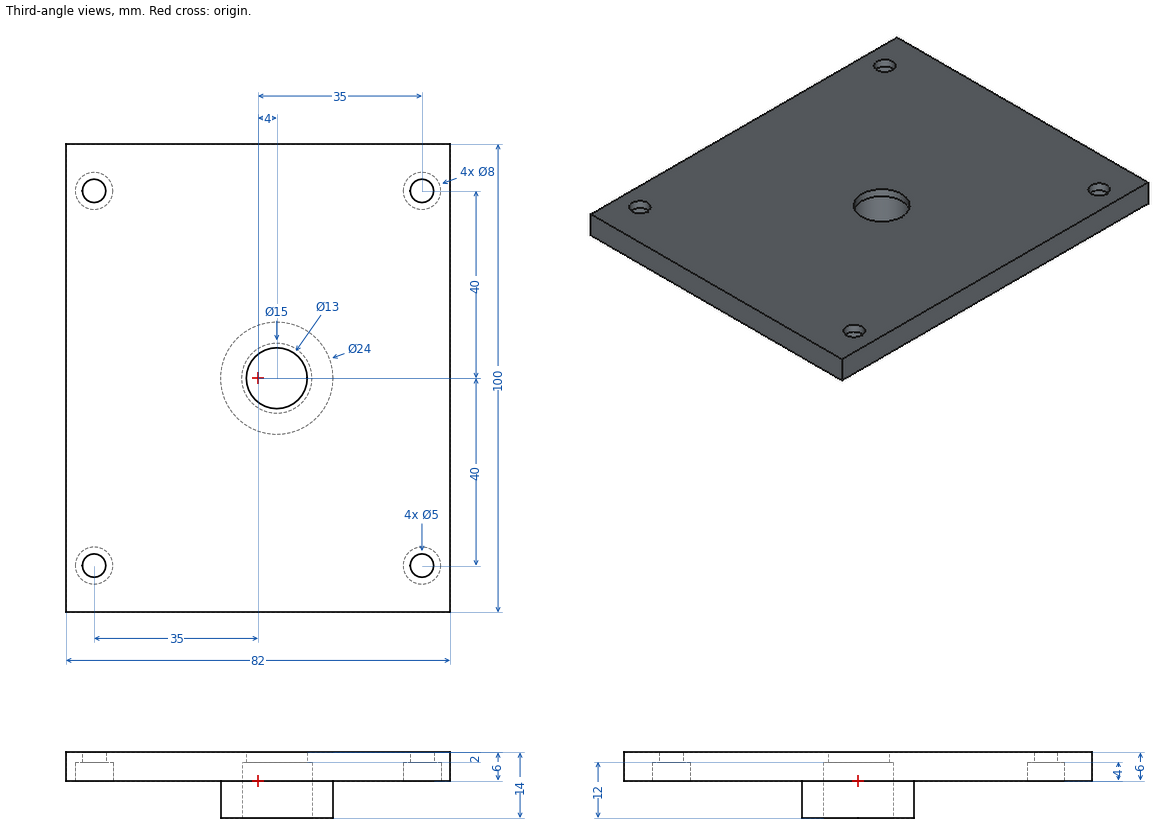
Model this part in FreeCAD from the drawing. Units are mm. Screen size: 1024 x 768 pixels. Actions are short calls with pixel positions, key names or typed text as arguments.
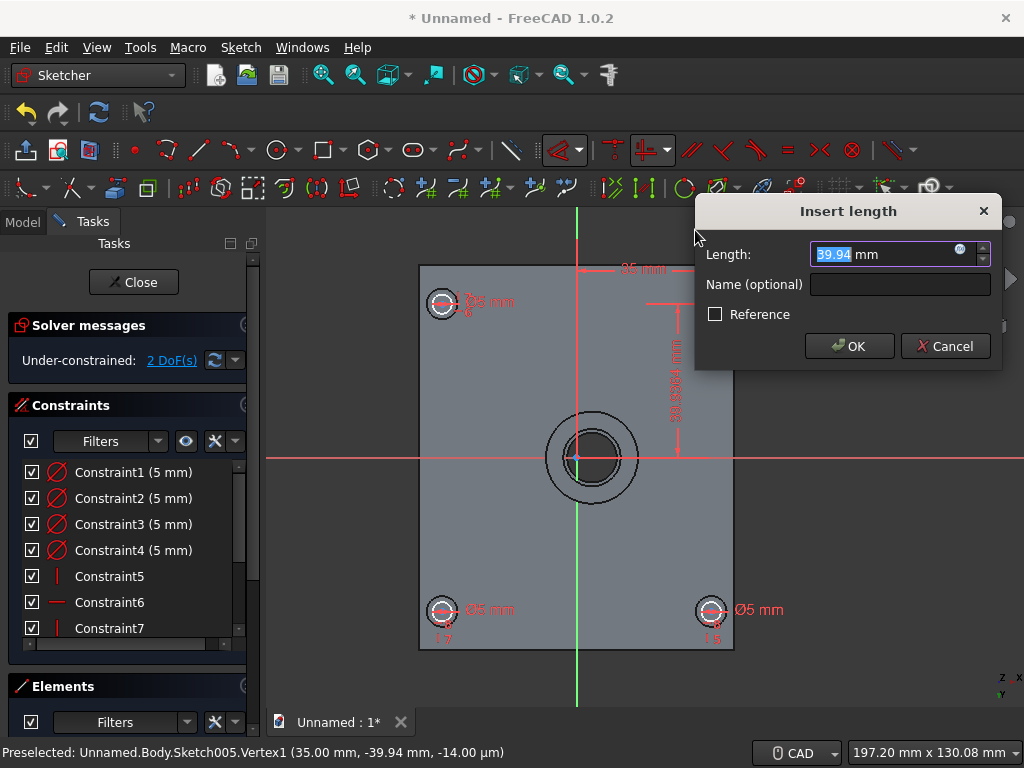
text(40)
key(Return)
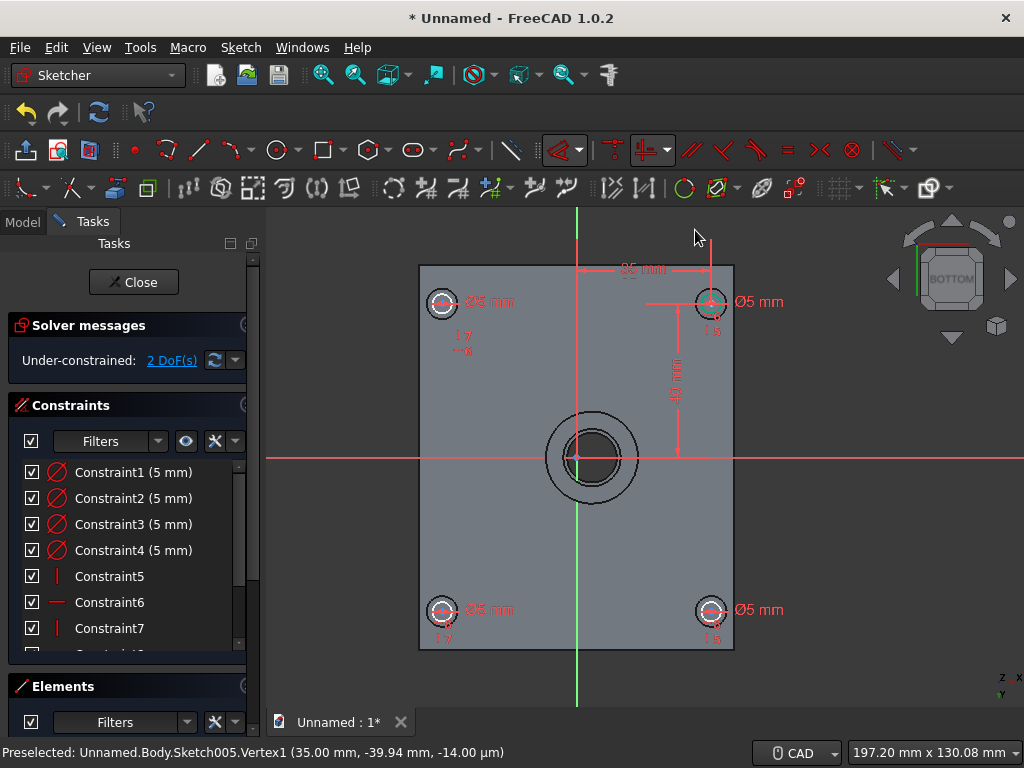
click(711, 612)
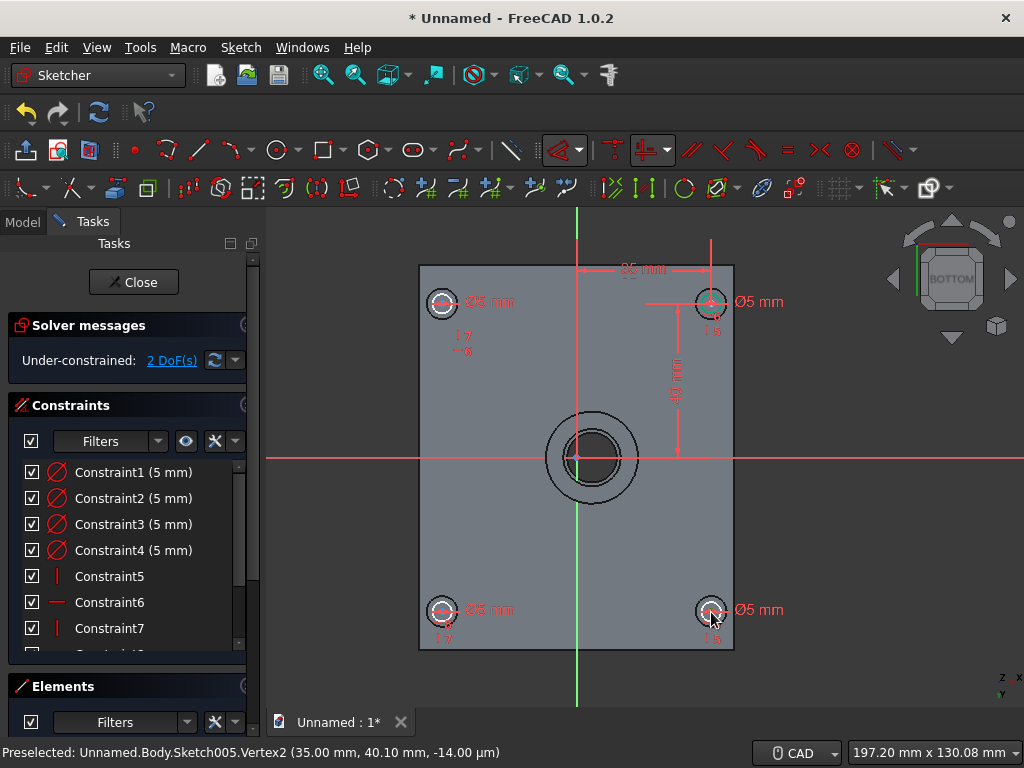
click(582, 150)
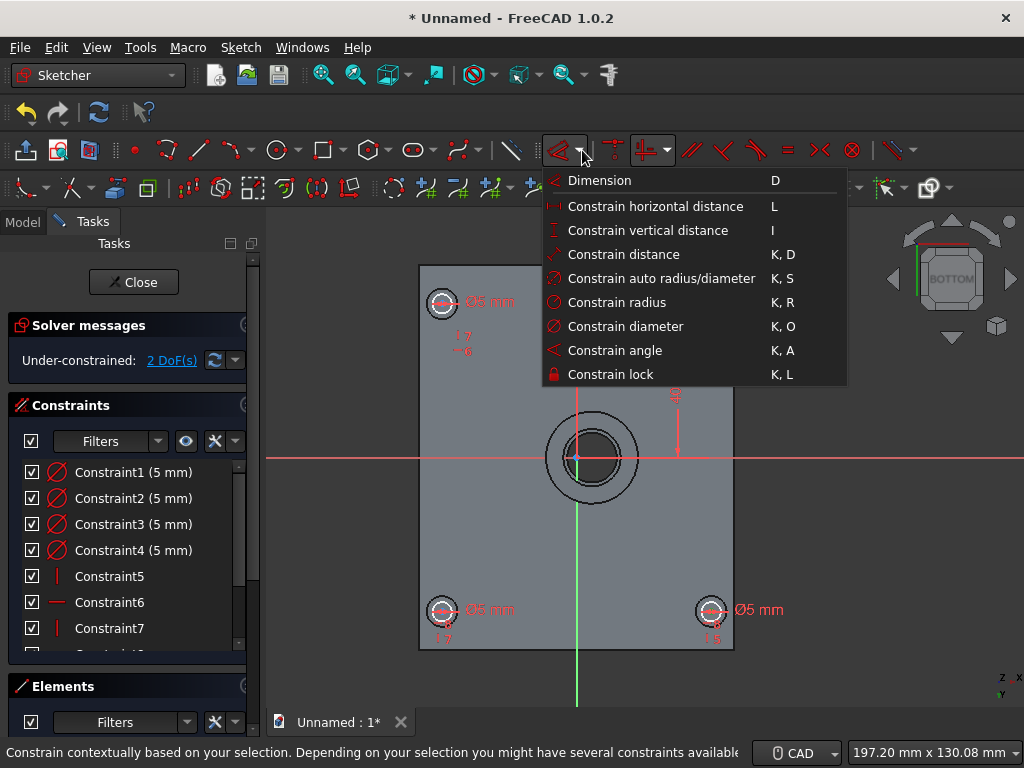
click(695, 230)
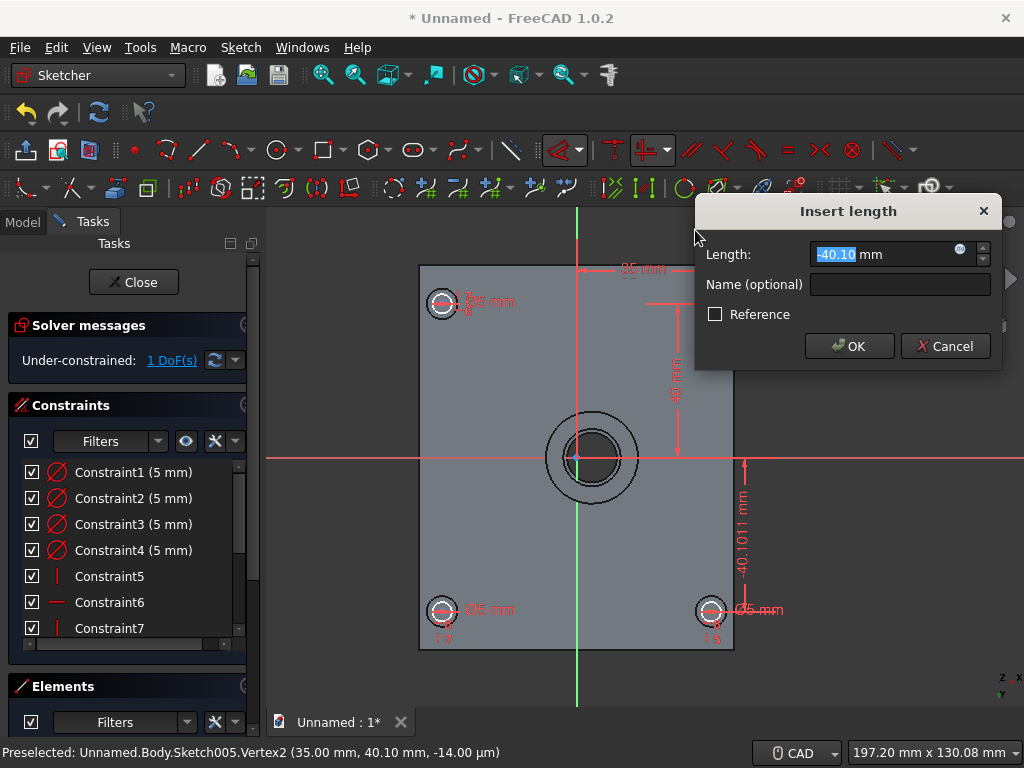
text(-40)
key(Return)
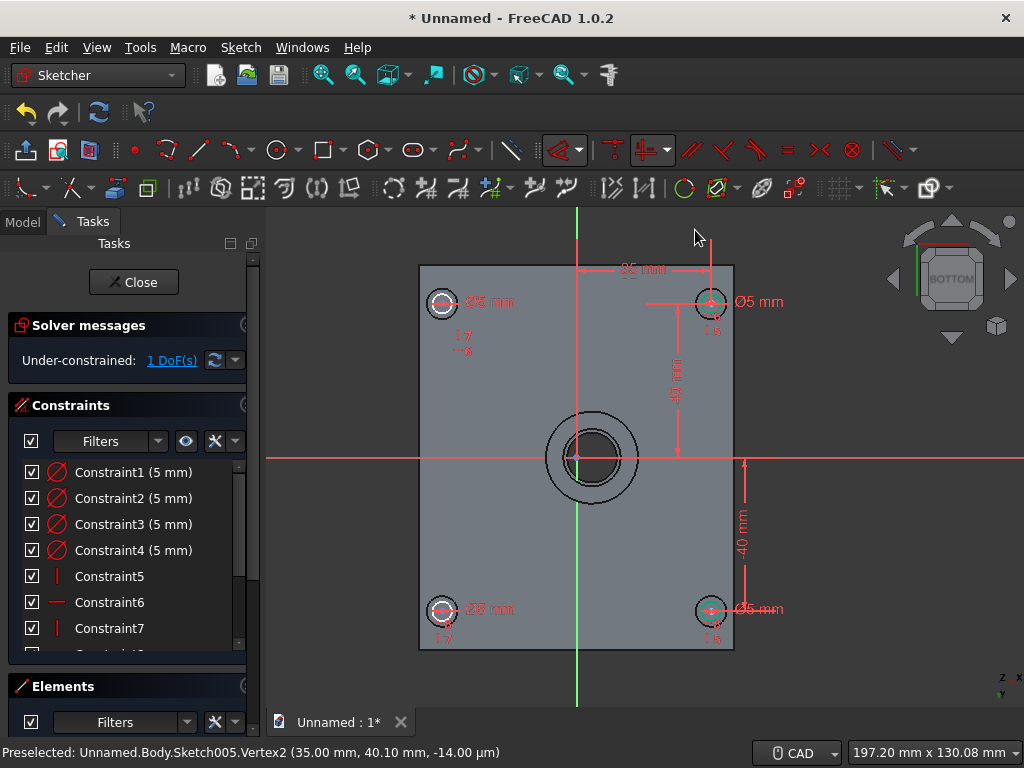
click(442, 304)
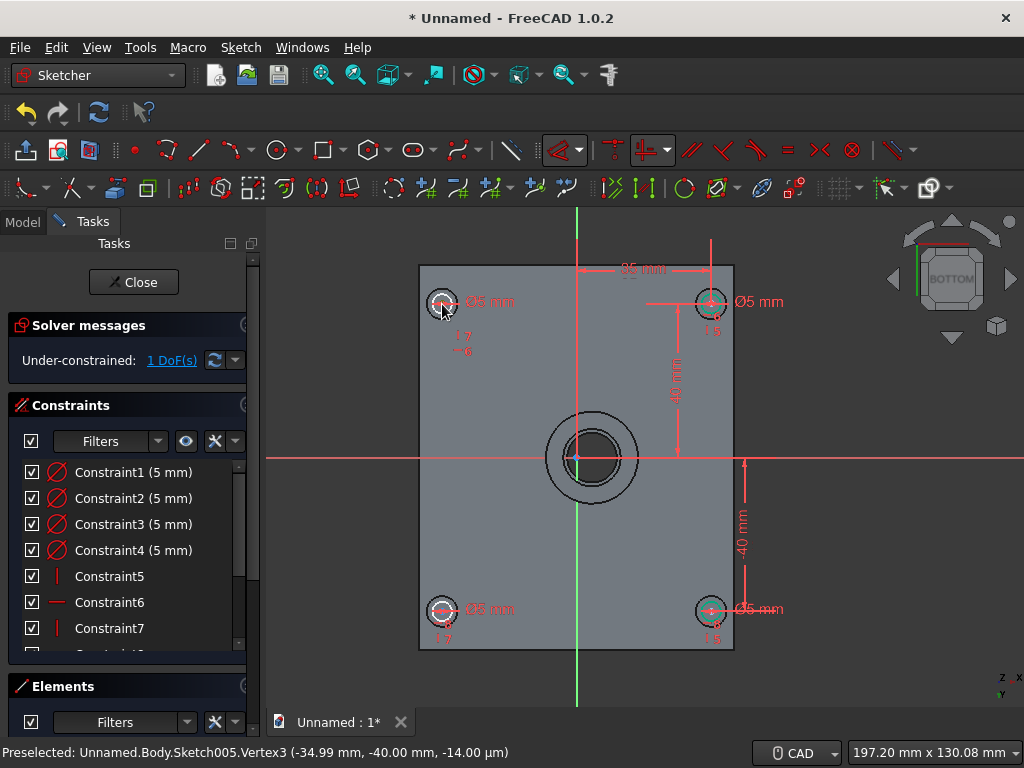
click(582, 150)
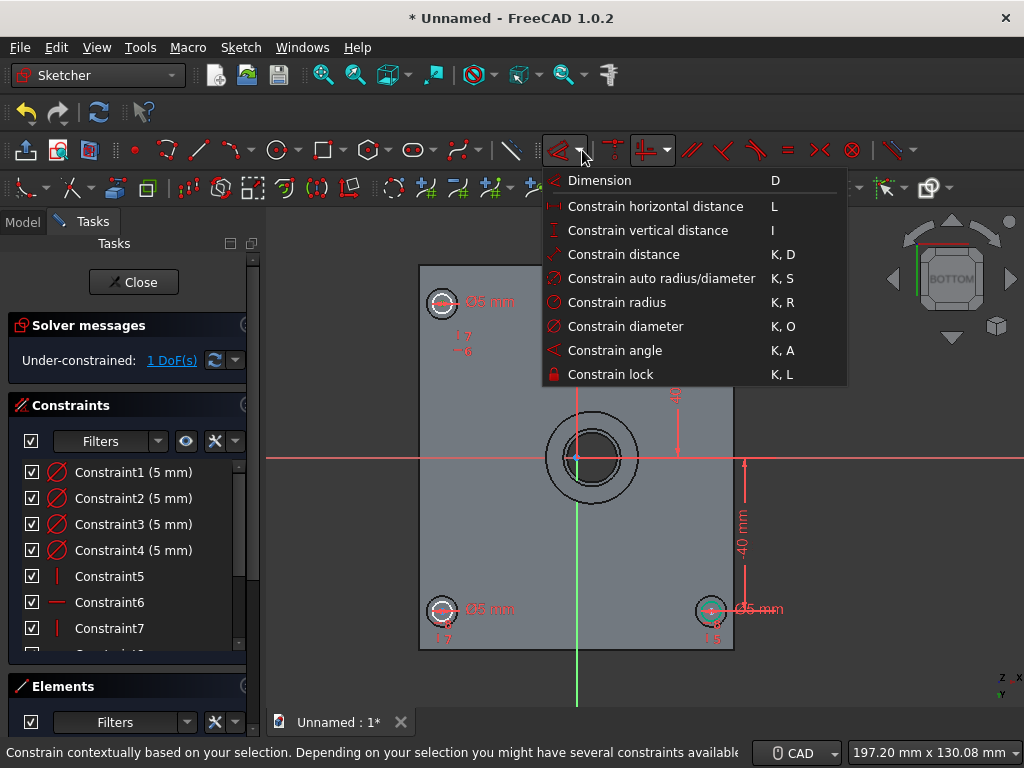
click(695, 206)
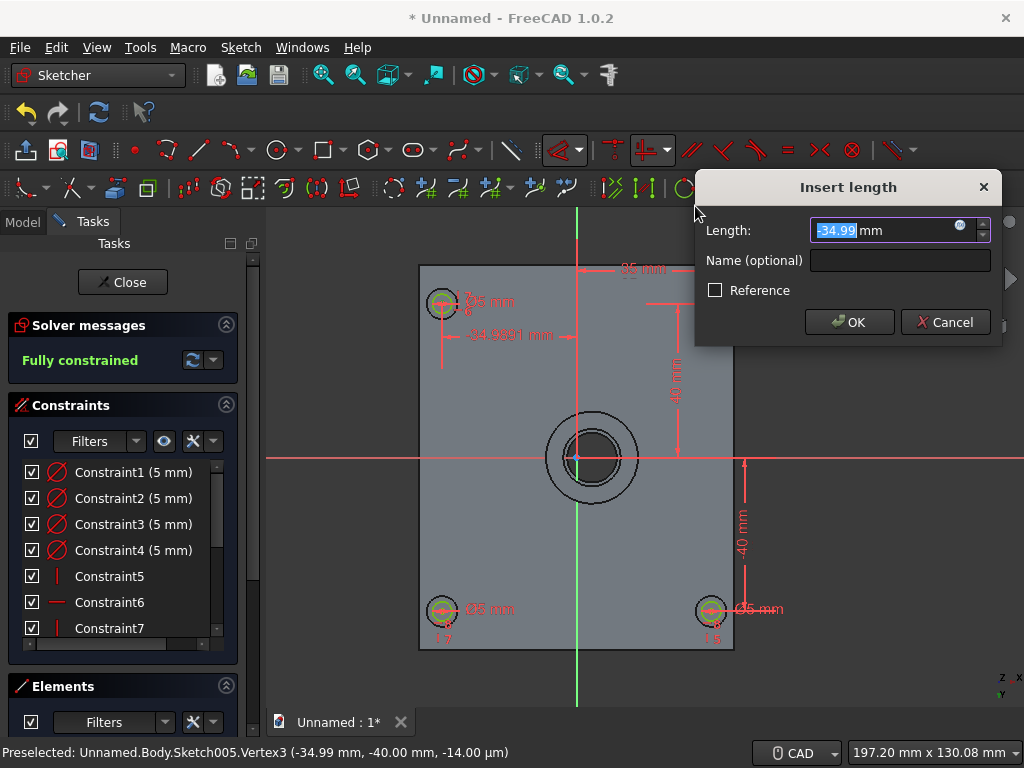
text(-35)
key(Return)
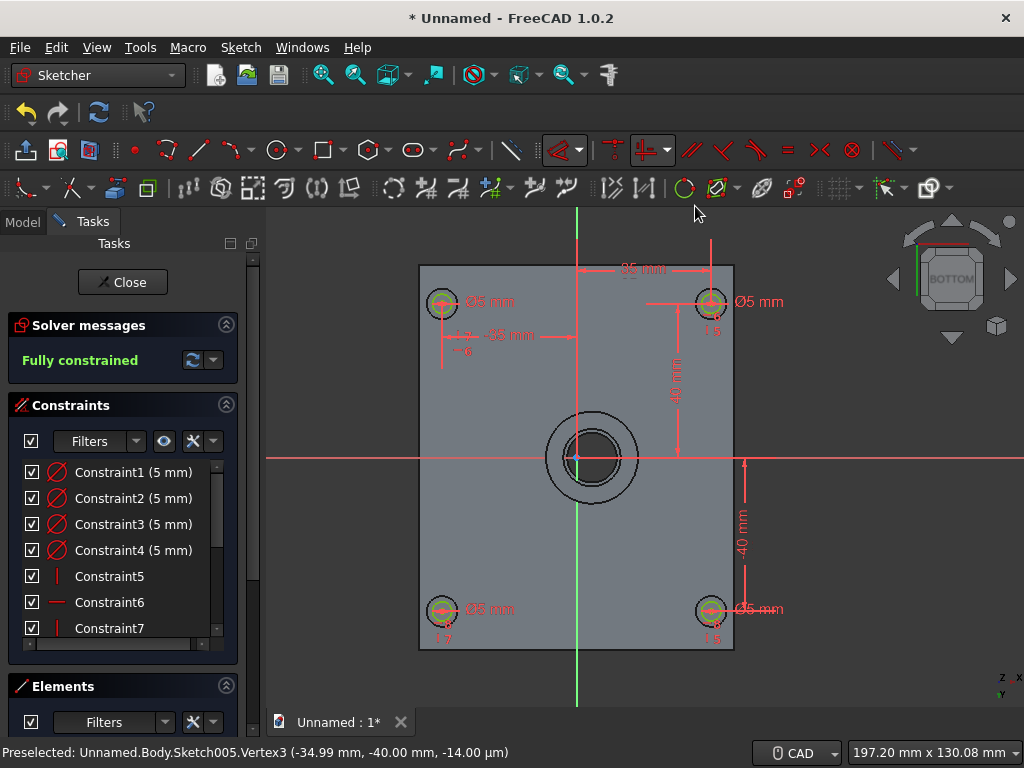
click(123, 282)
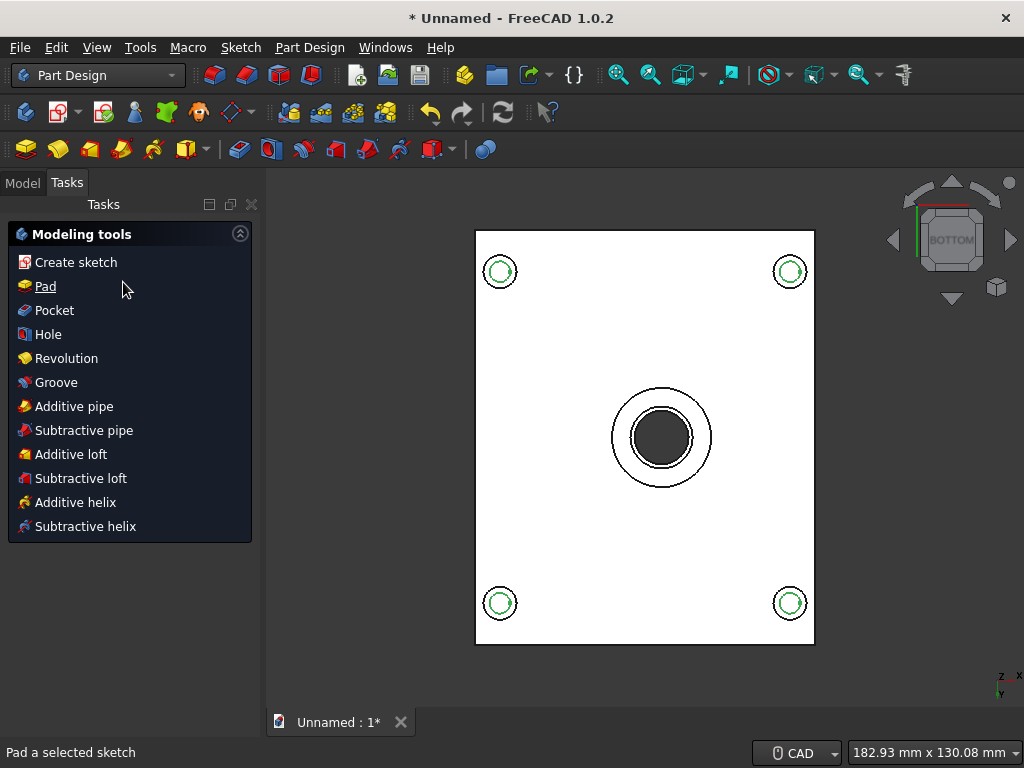
click(240, 150)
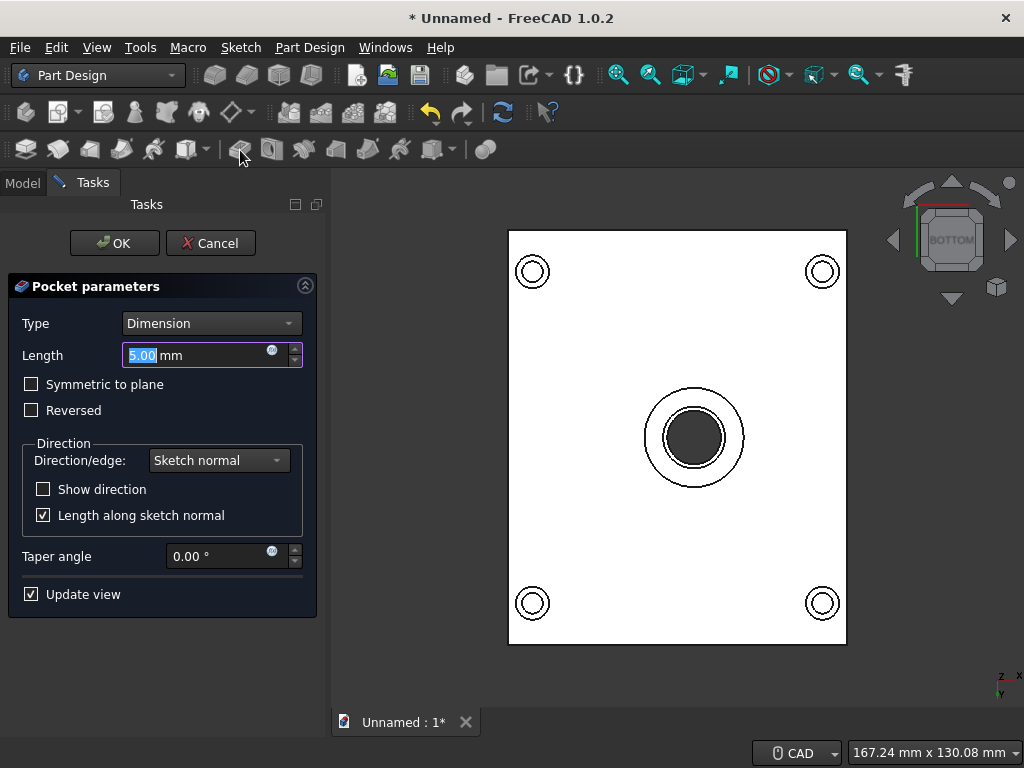
text(6)
key(Tab)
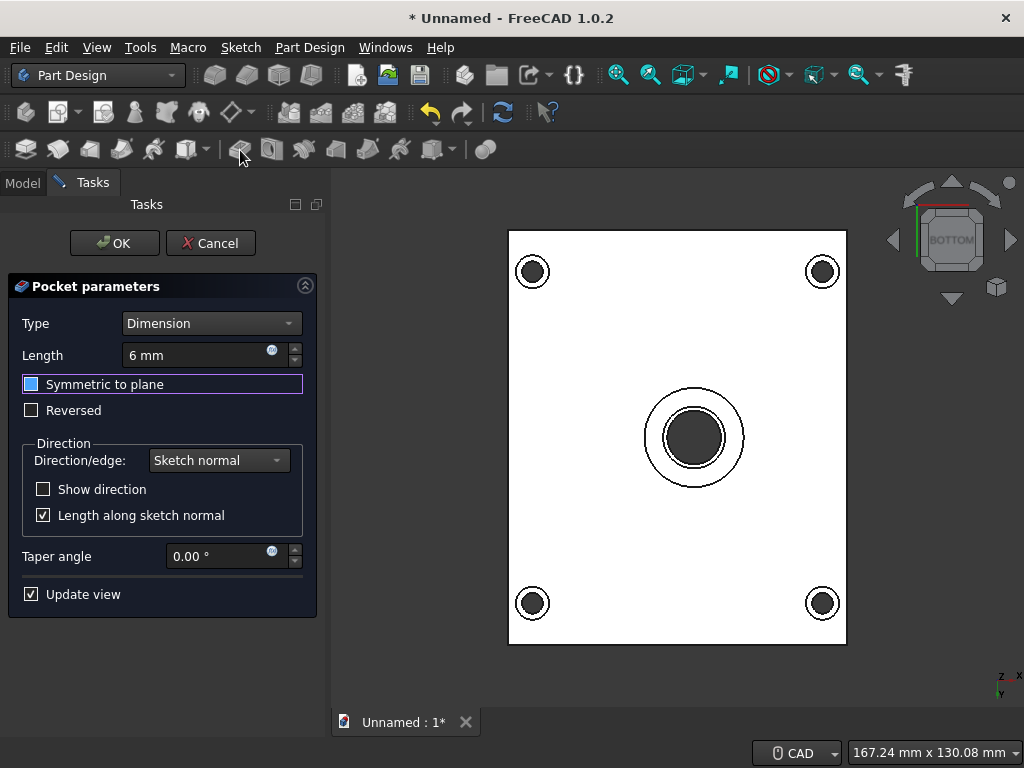
click(115, 243)